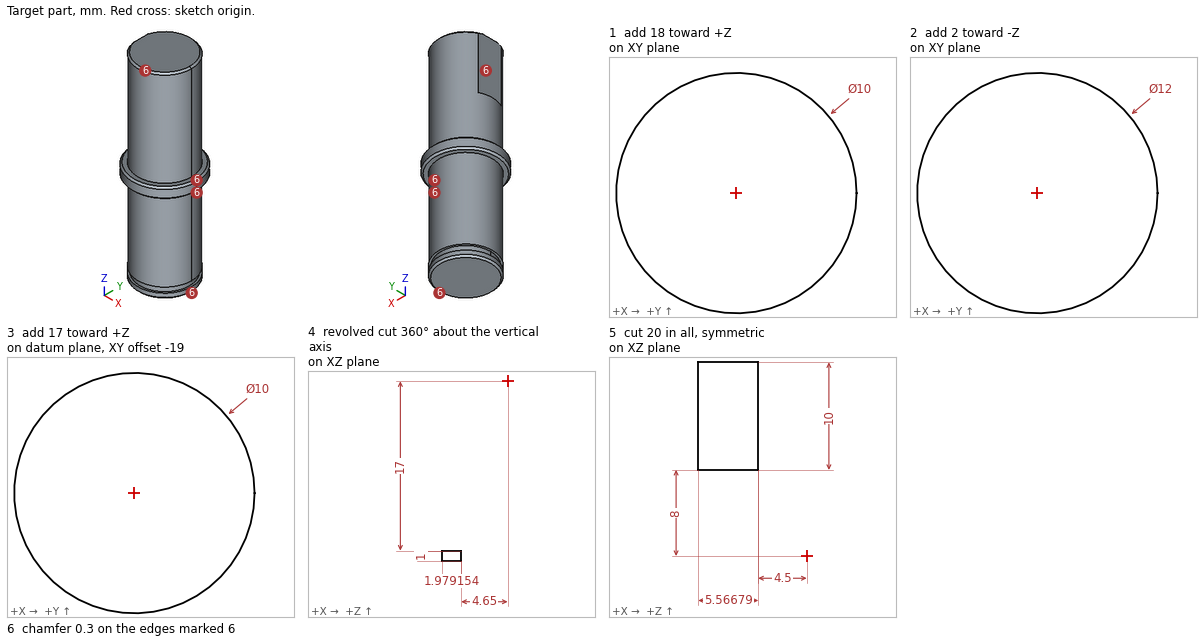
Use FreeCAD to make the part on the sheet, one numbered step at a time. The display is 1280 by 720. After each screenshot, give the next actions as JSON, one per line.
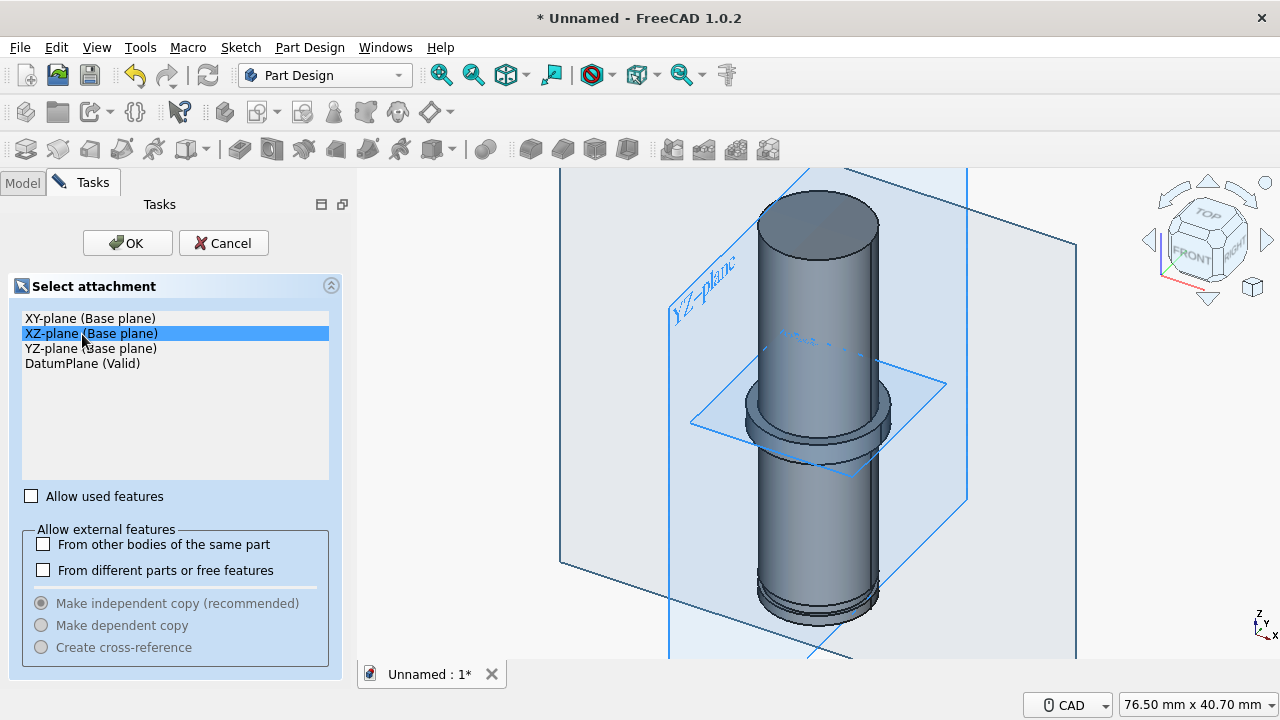
{"action": "left_click", "coordinate": [128, 243]}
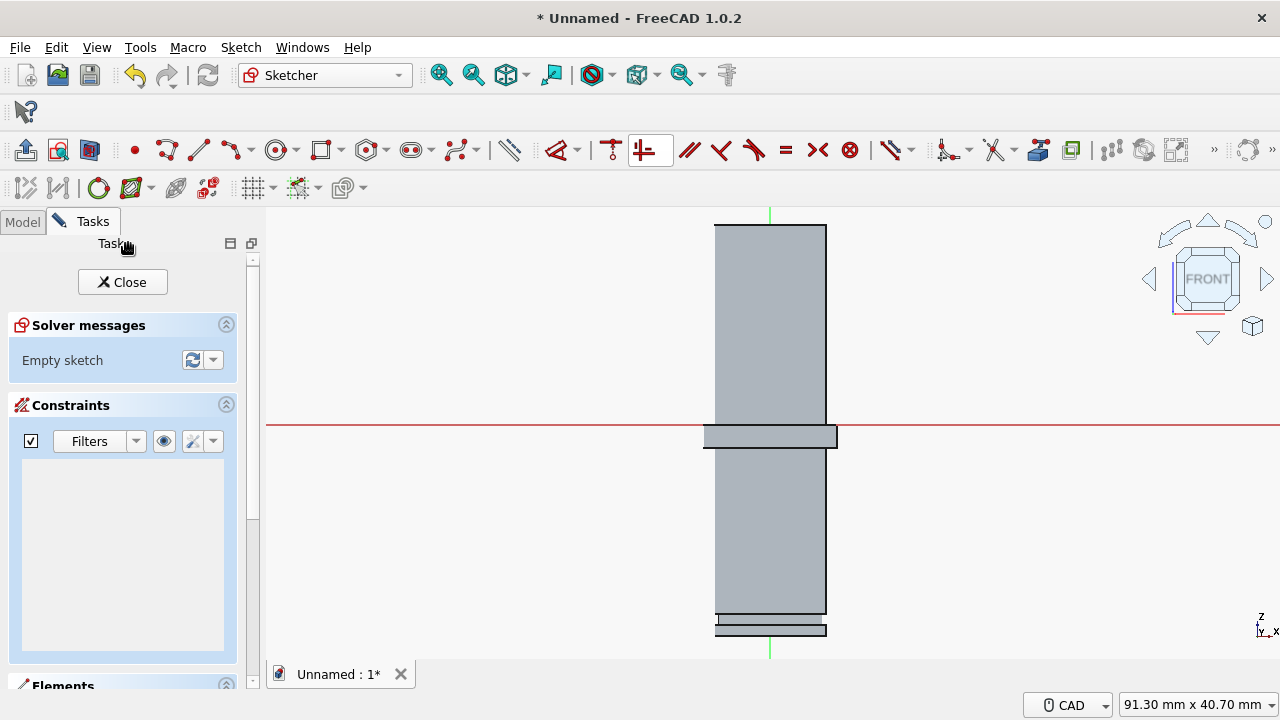
{"action": "left_click", "coordinate": [90, 150]}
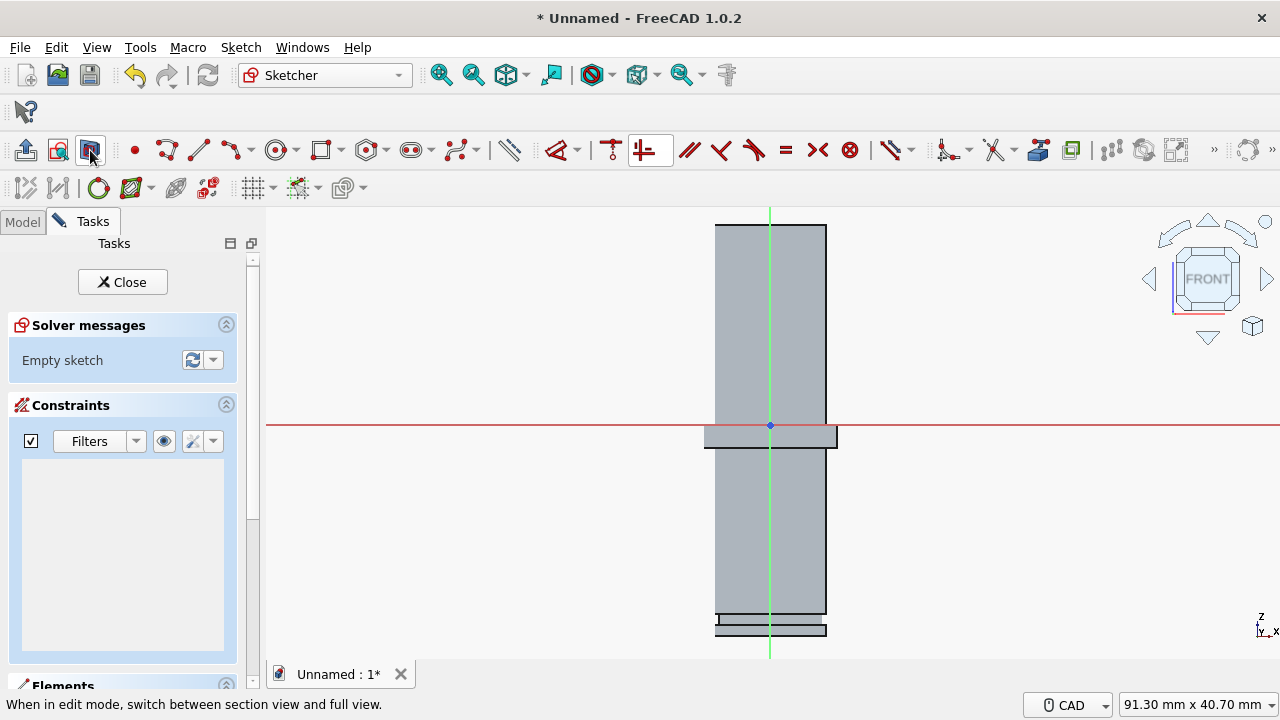
{"action": "scroll", "coordinate": [660, 631], "scroll_direction": "down", "scroll_amount": 1}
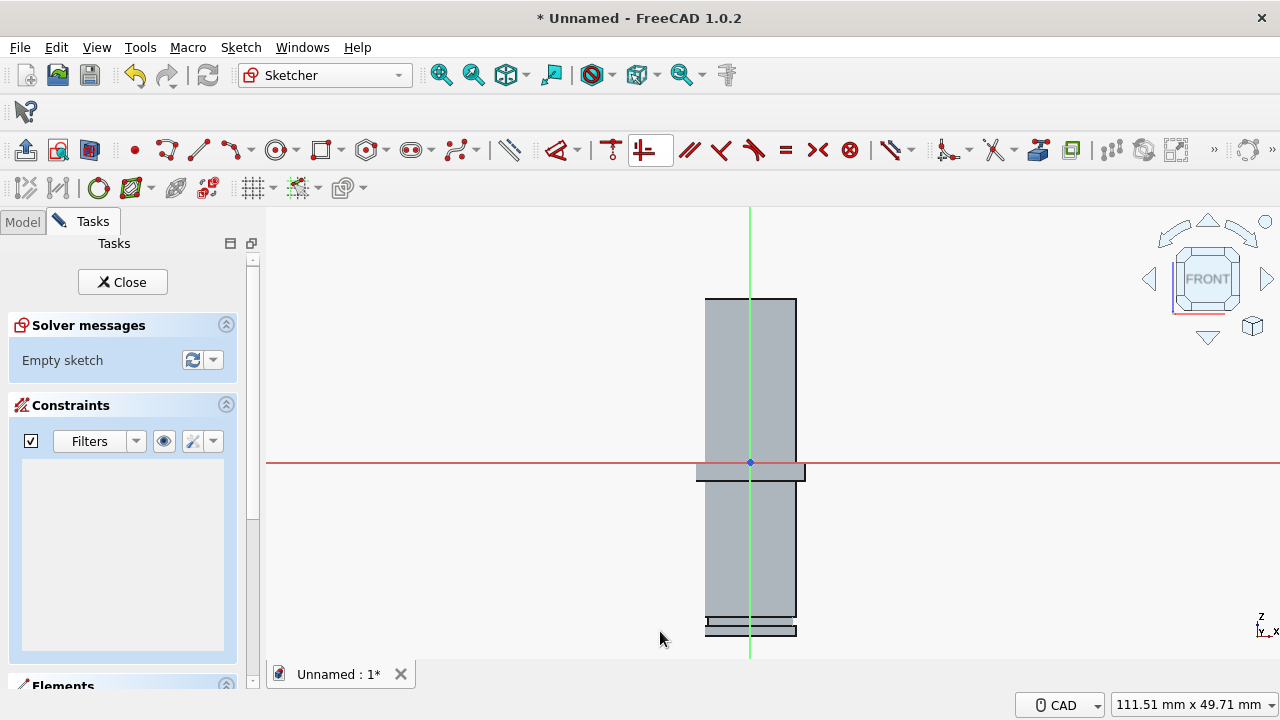
{"action": "scroll", "coordinate": [705, 318], "scroll_direction": "up", "scroll_amount": 3}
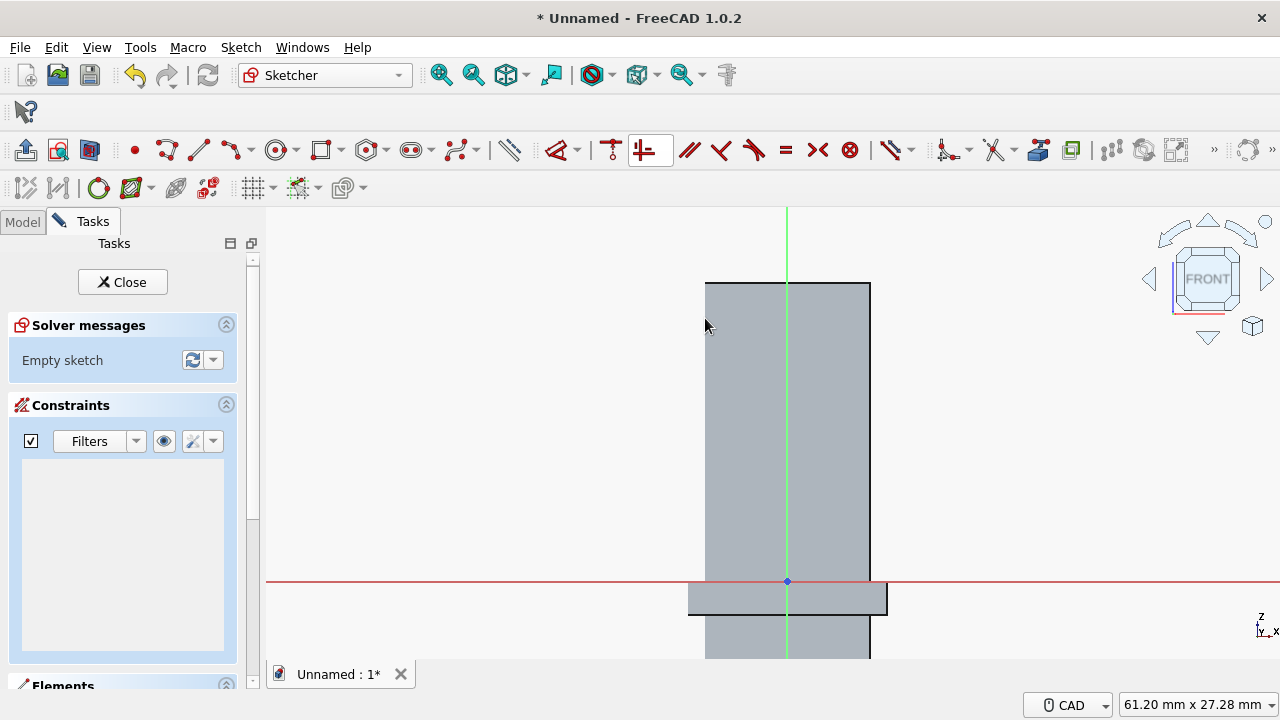
{"action": "left_click", "coordinate": [322, 150]}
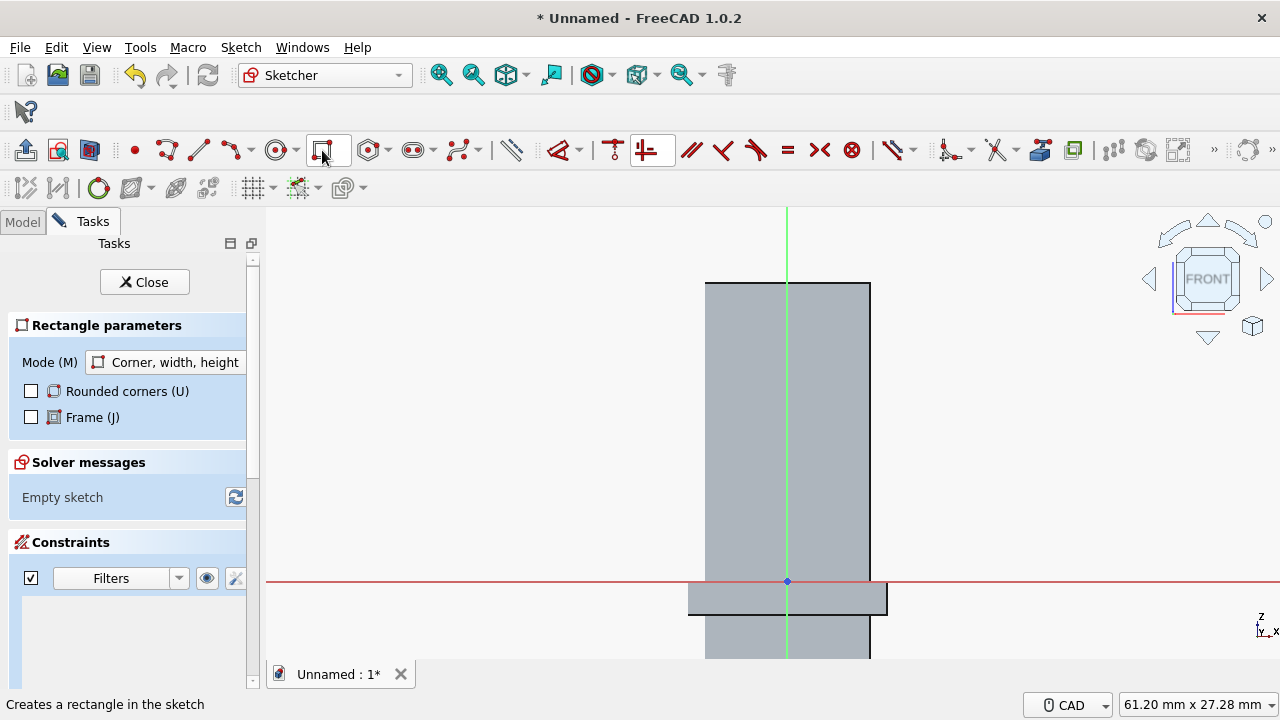
{"action": "left_click", "coordinate": [620, 283]}
{"action": "mouse_move", "coordinate": [713, 449]}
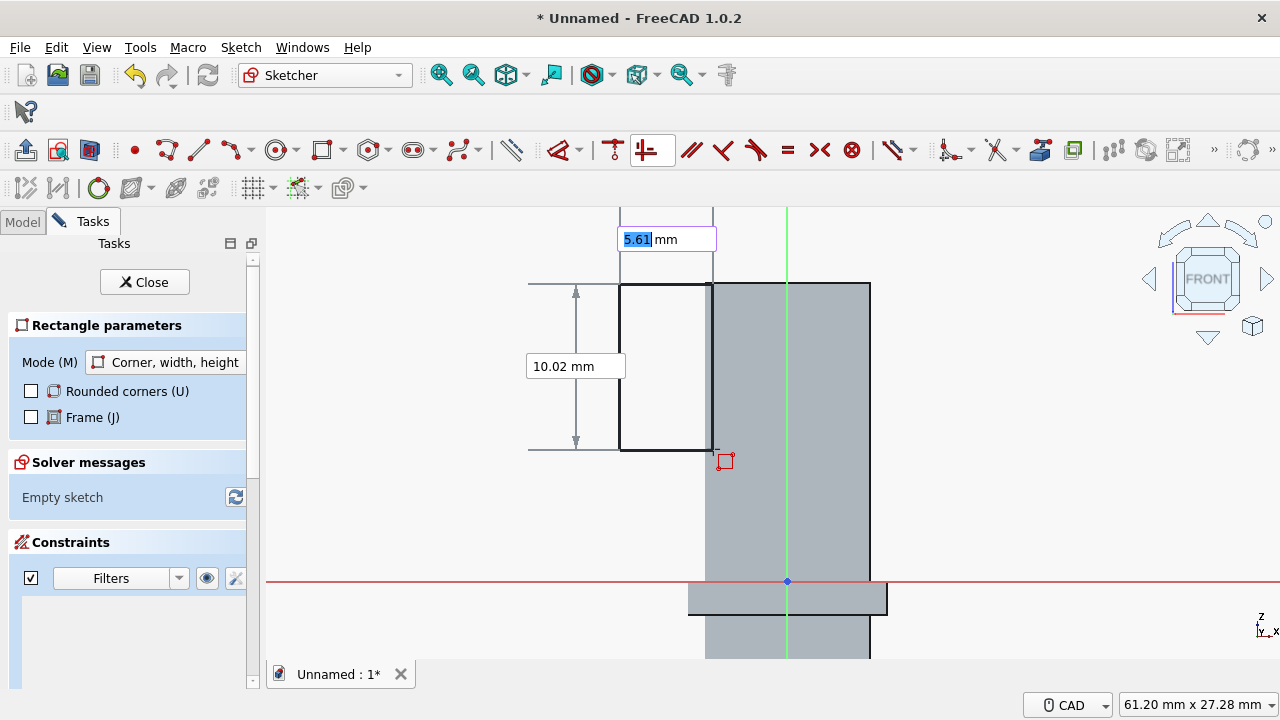
{"action": "type", "text": "5.56679"}
{"action": "key", "text": "Tab"}
{"action": "type", "text": "10"}
{"action": "key", "text": "Return"}
{"action": "key", "text": "Escape"}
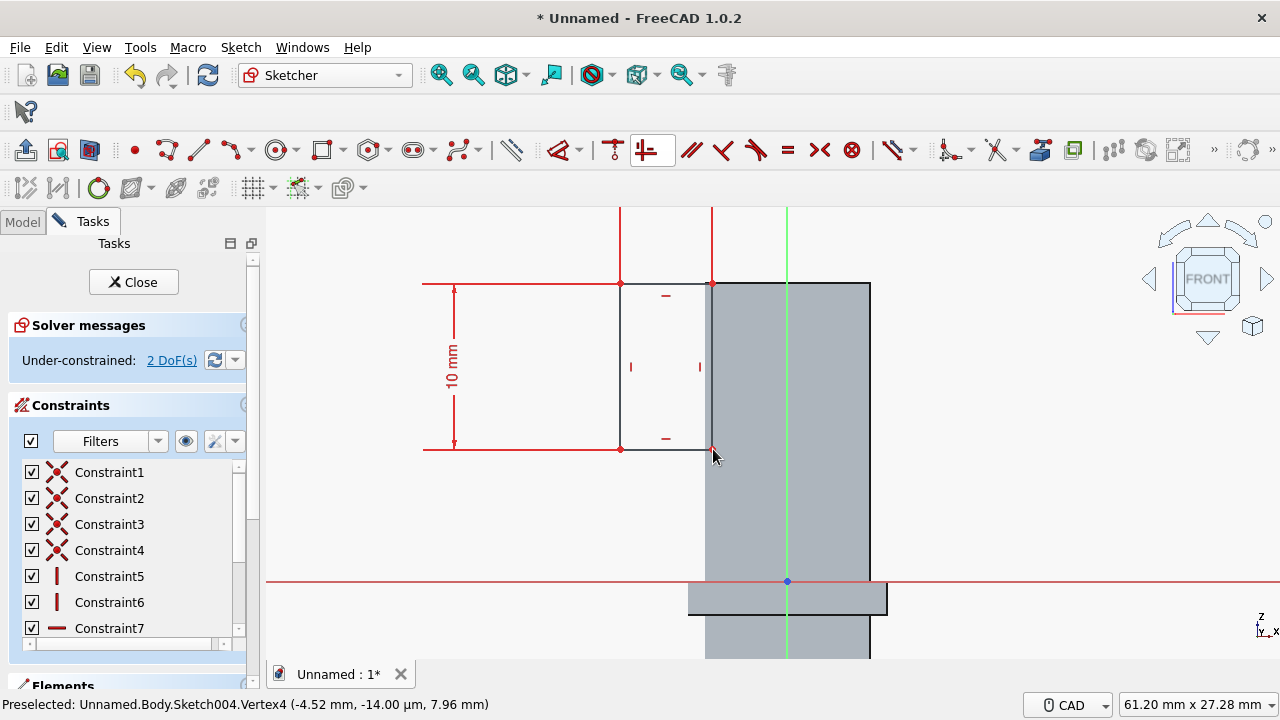
{"action": "left_click", "coordinate": [558, 150]}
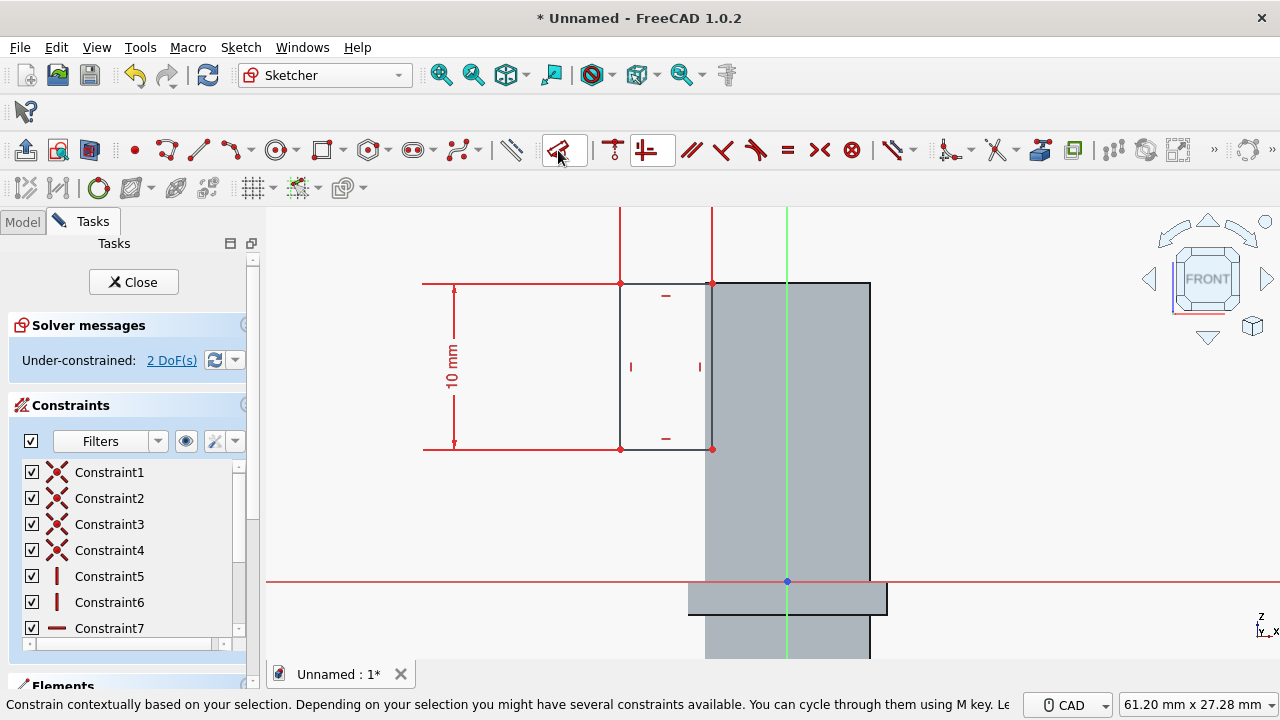
{"action": "left_click", "coordinate": [620, 450]}
{"action": "left_click", "coordinate": [586, 516]}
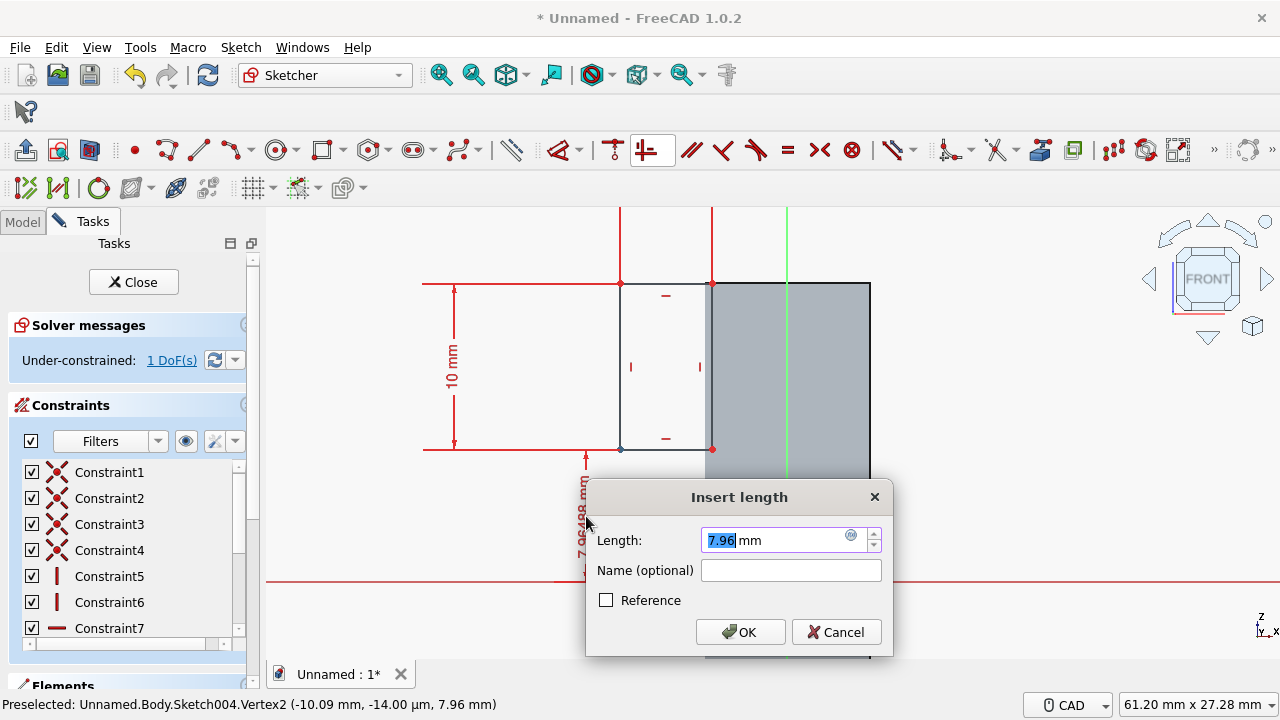
{"action": "type", "text": "8"}
{"action": "key", "text": "Return"}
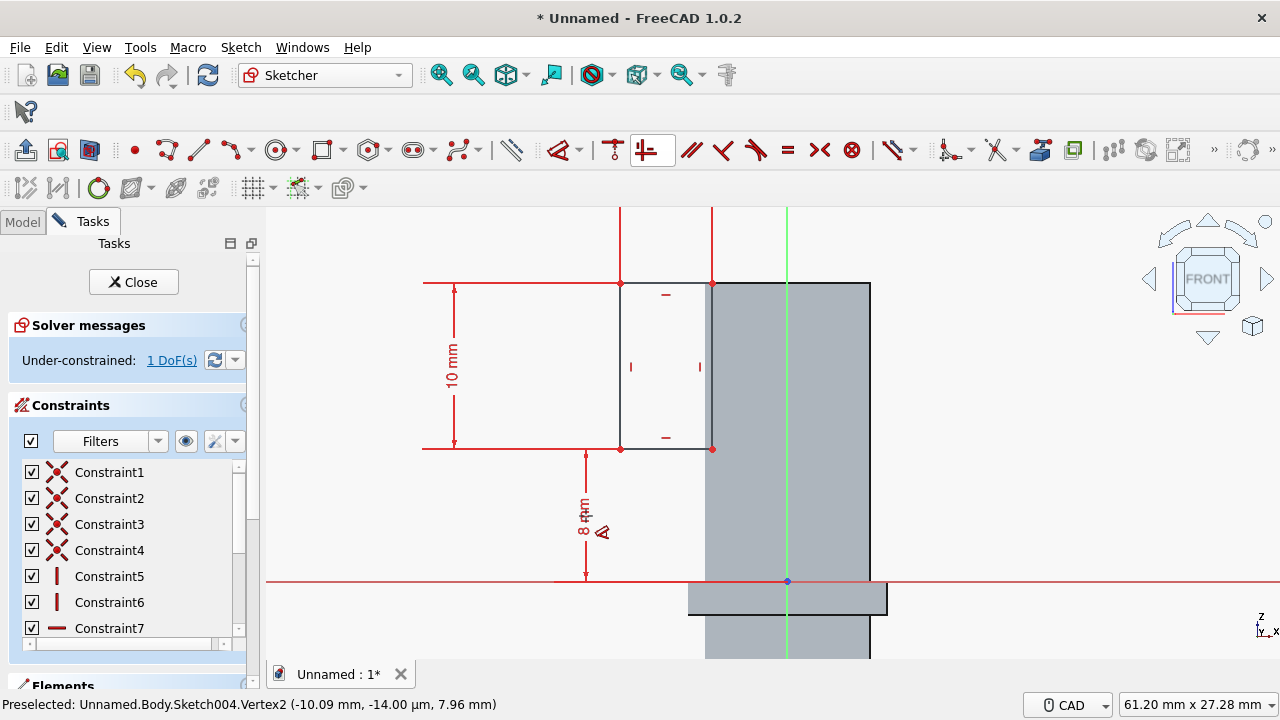
{"action": "left_click", "coordinate": [712, 449]}
{"action": "left_click", "coordinate": [750, 616]}